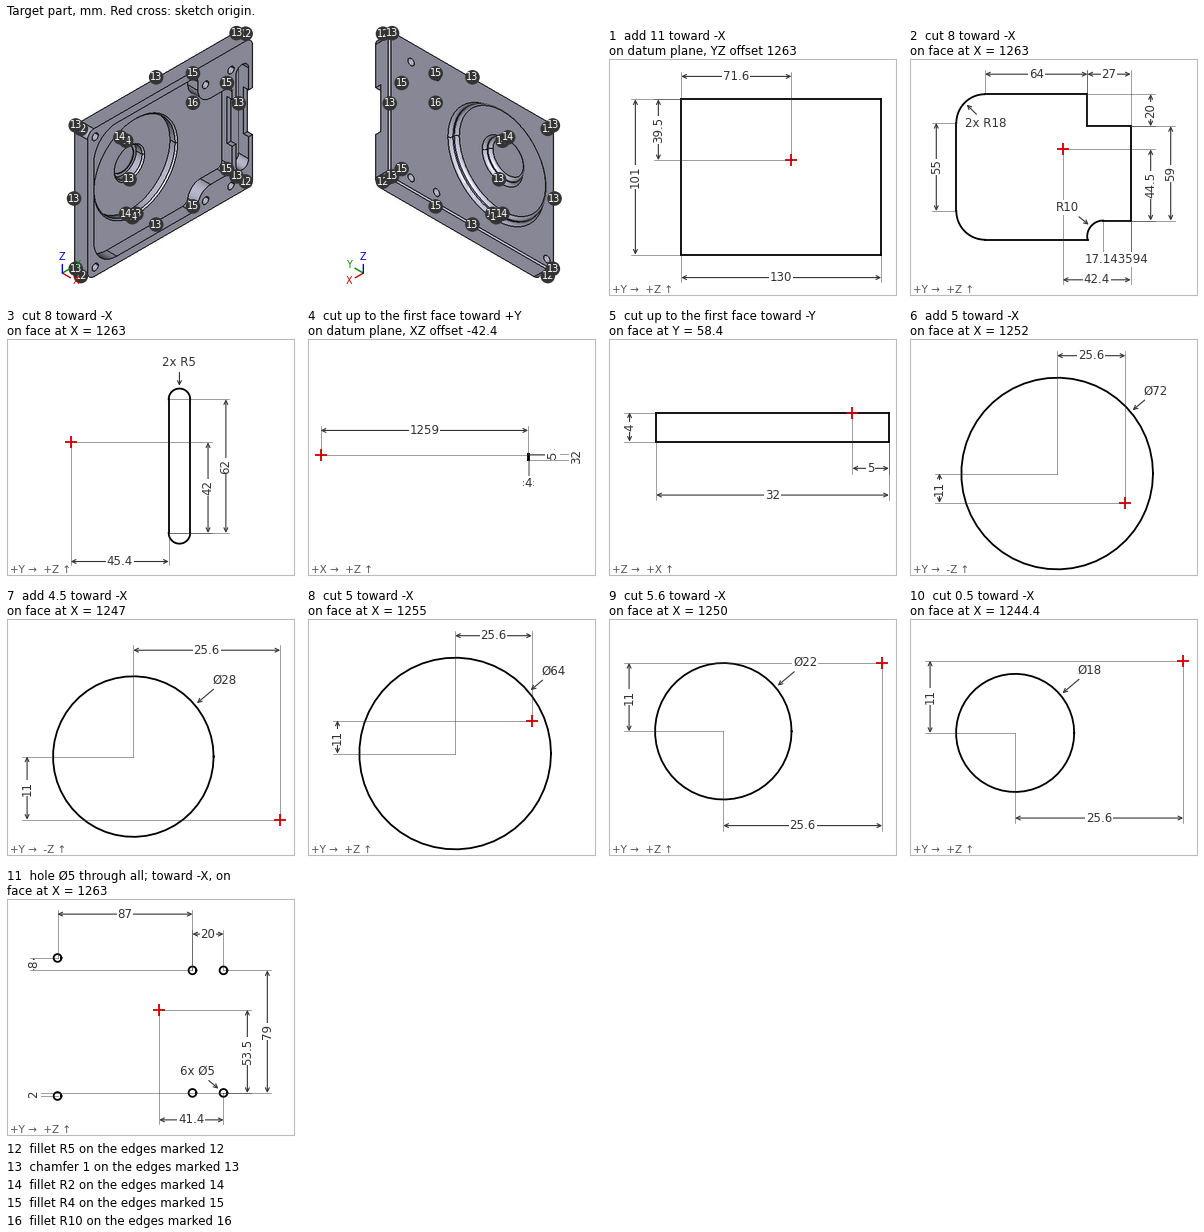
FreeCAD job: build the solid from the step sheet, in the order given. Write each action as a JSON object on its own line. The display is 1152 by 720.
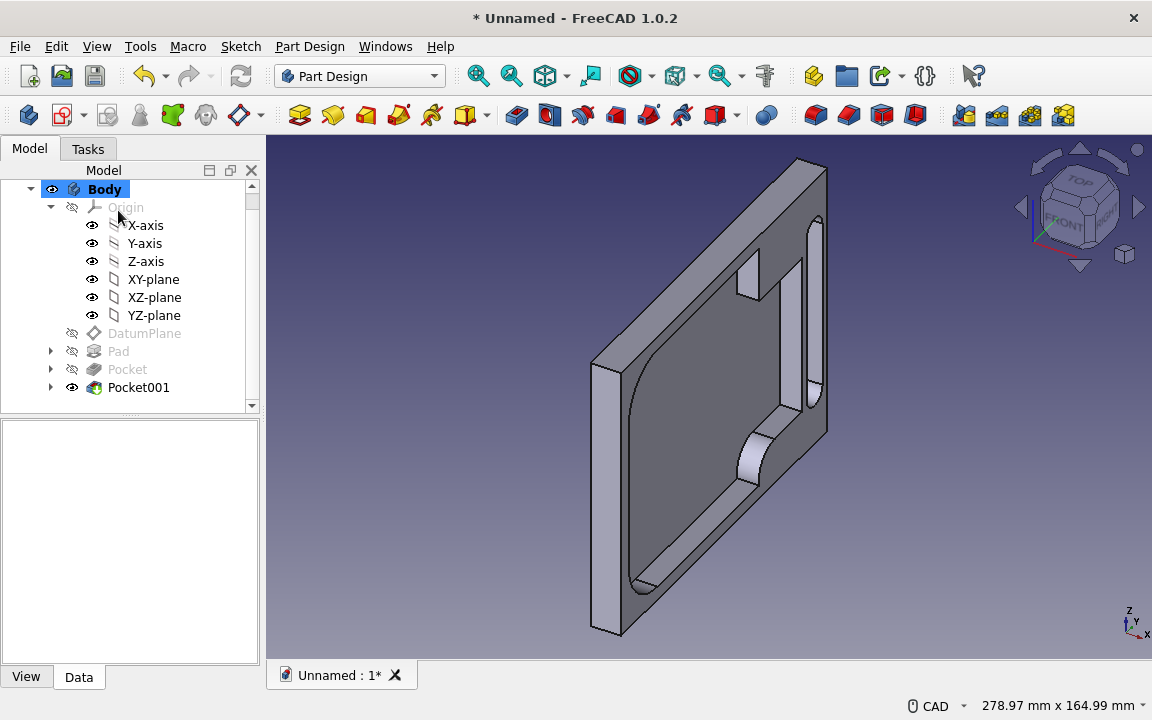
{"action": "left_click", "coordinate": [137, 297]}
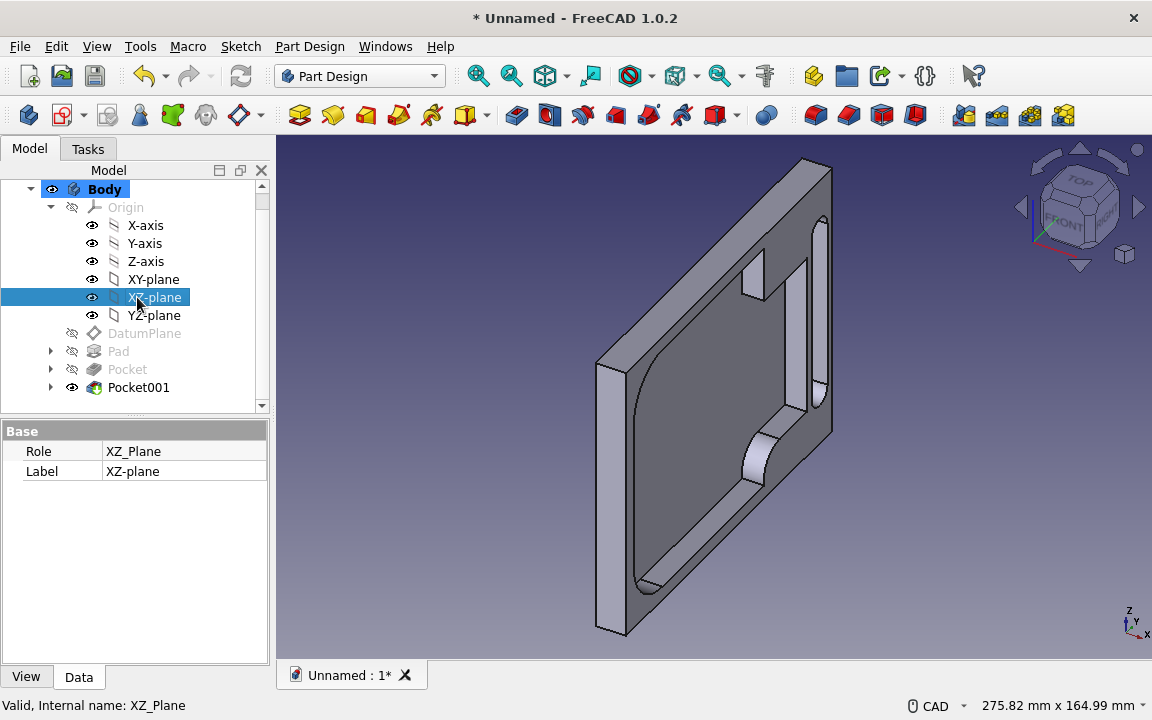
{"action": "left_click", "coordinate": [238, 116]}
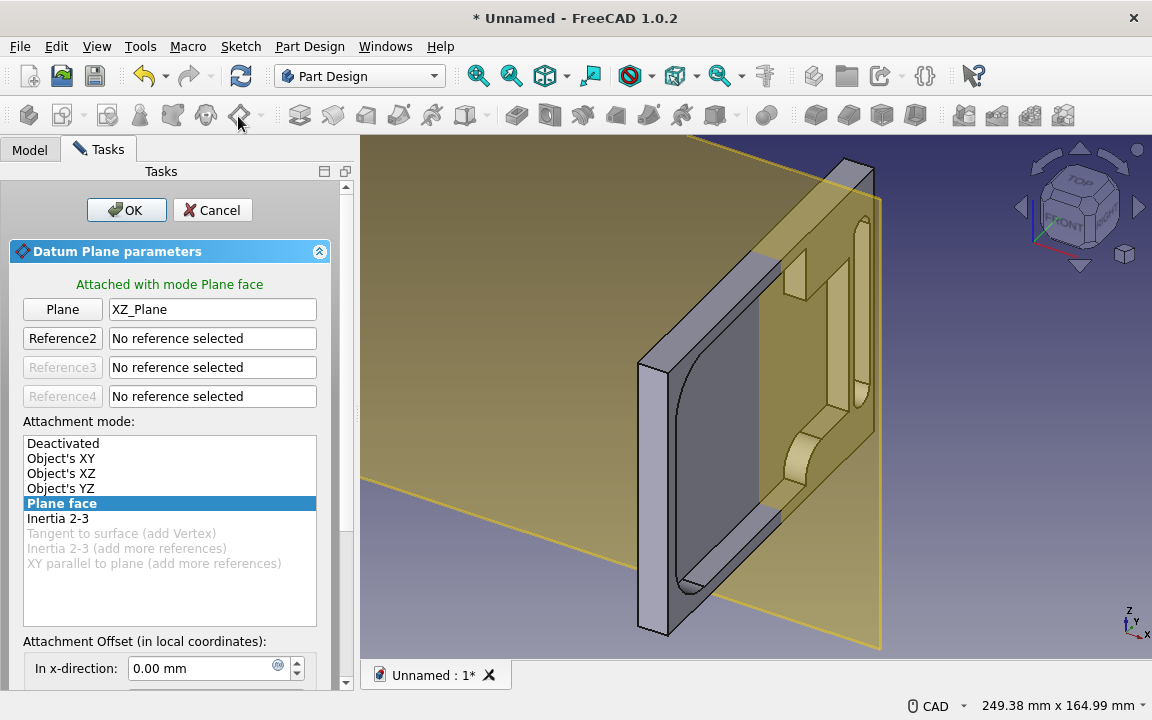
{"action": "scroll", "coordinate": [346, 436], "scroll_direction": "down", "scroll_amount": 2}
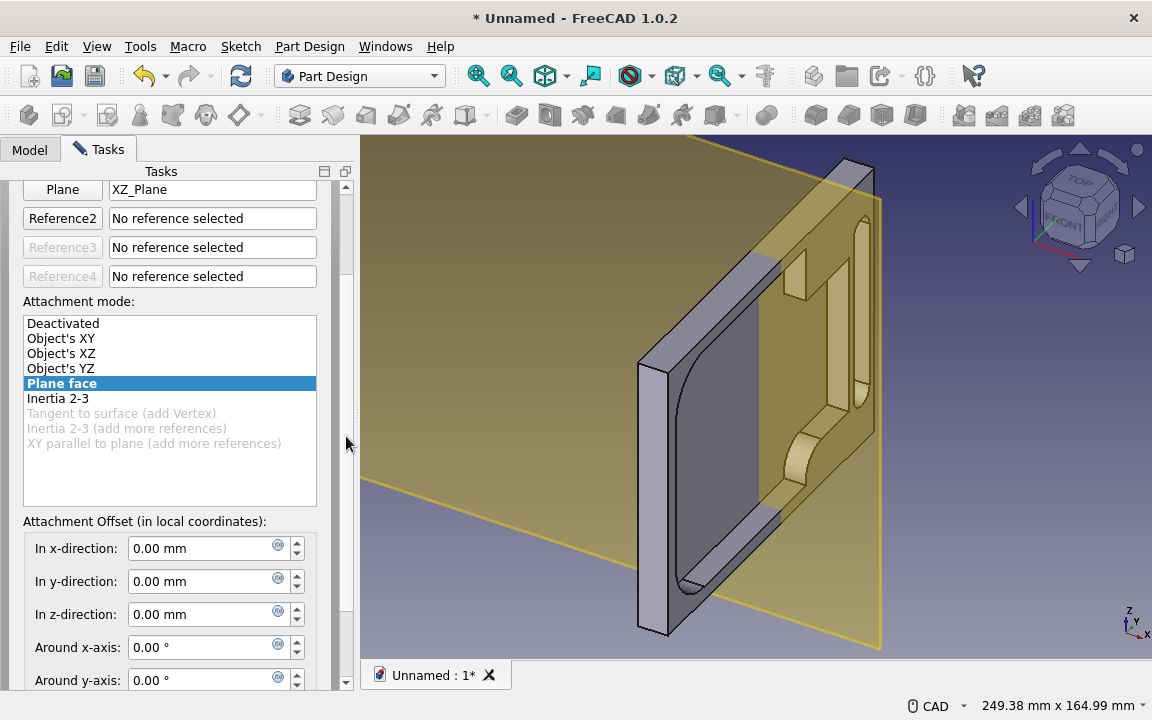
{"action": "triple_click", "coordinate": [210, 614]}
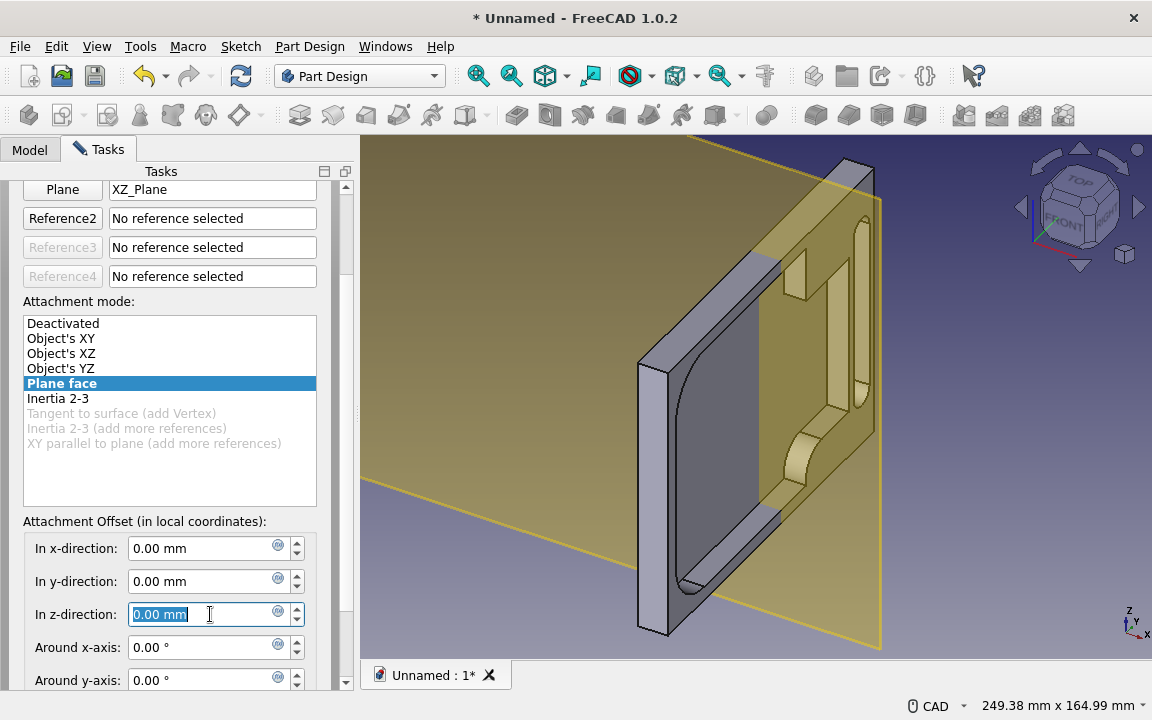
{"action": "type", "text": "-42.4"}
{"action": "key", "text": "Tab"}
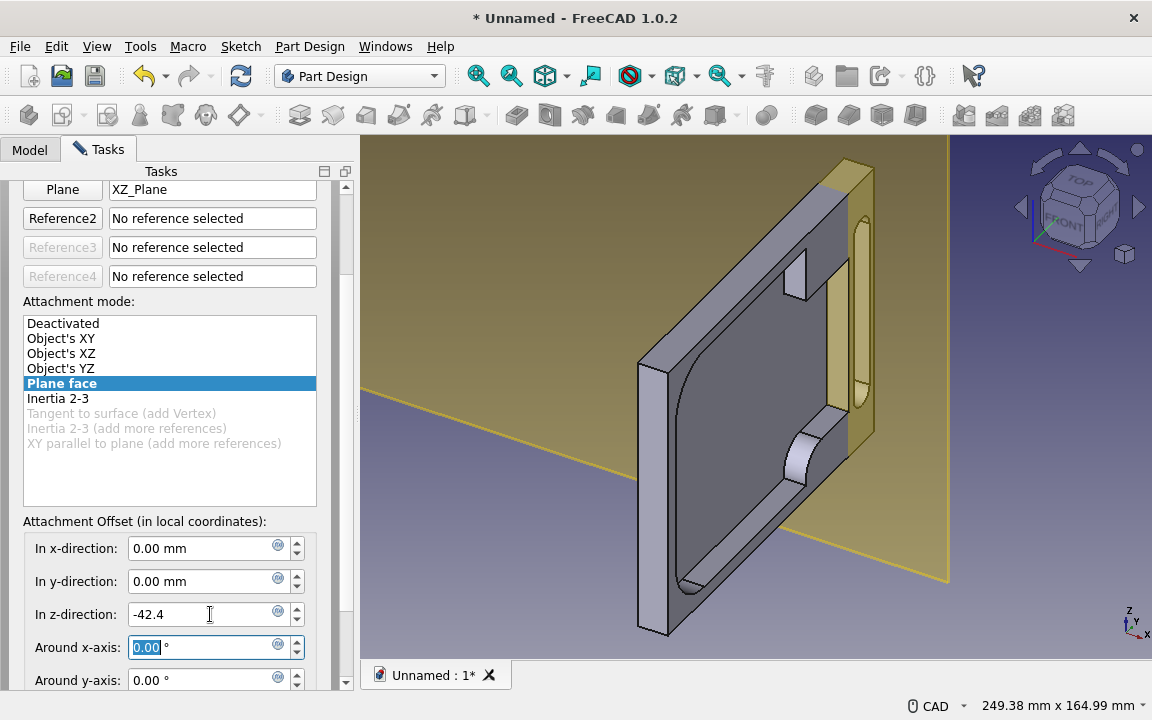
{"action": "scroll", "coordinate": [346, 436], "scroll_direction": "up", "scroll_amount": 3}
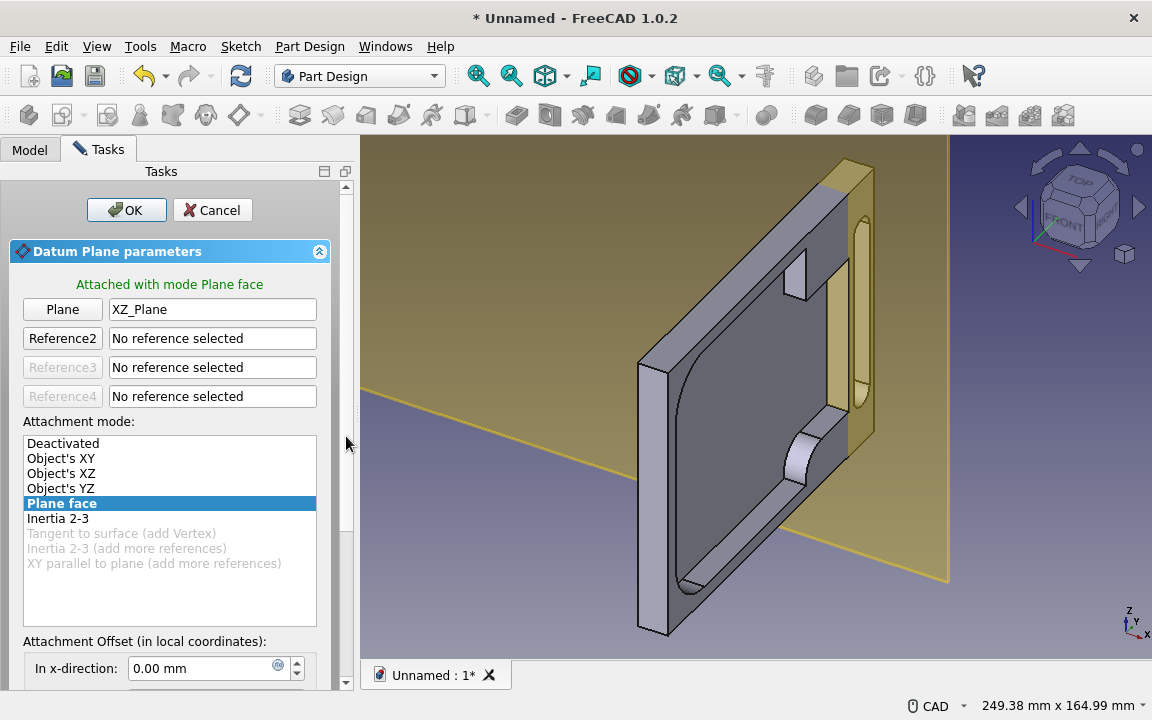
{"action": "left_click", "coordinate": [127, 210]}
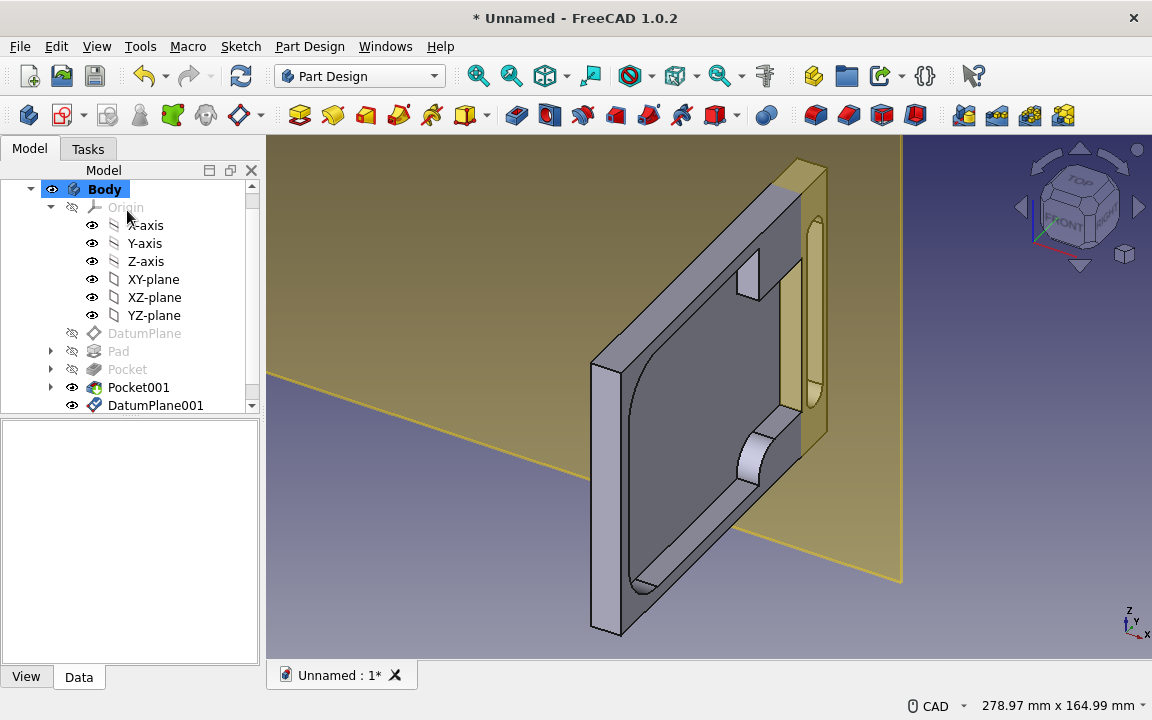
{"action": "left_click", "coordinate": [117, 405]}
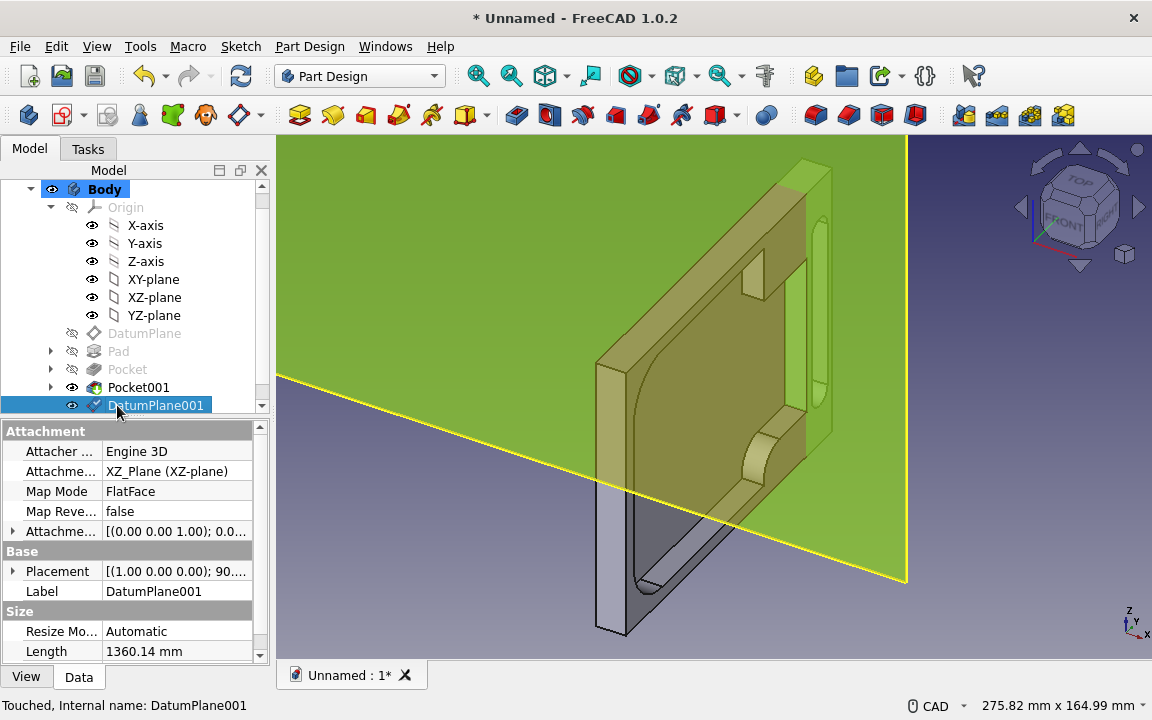
{"action": "left_click", "coordinate": [62, 116]}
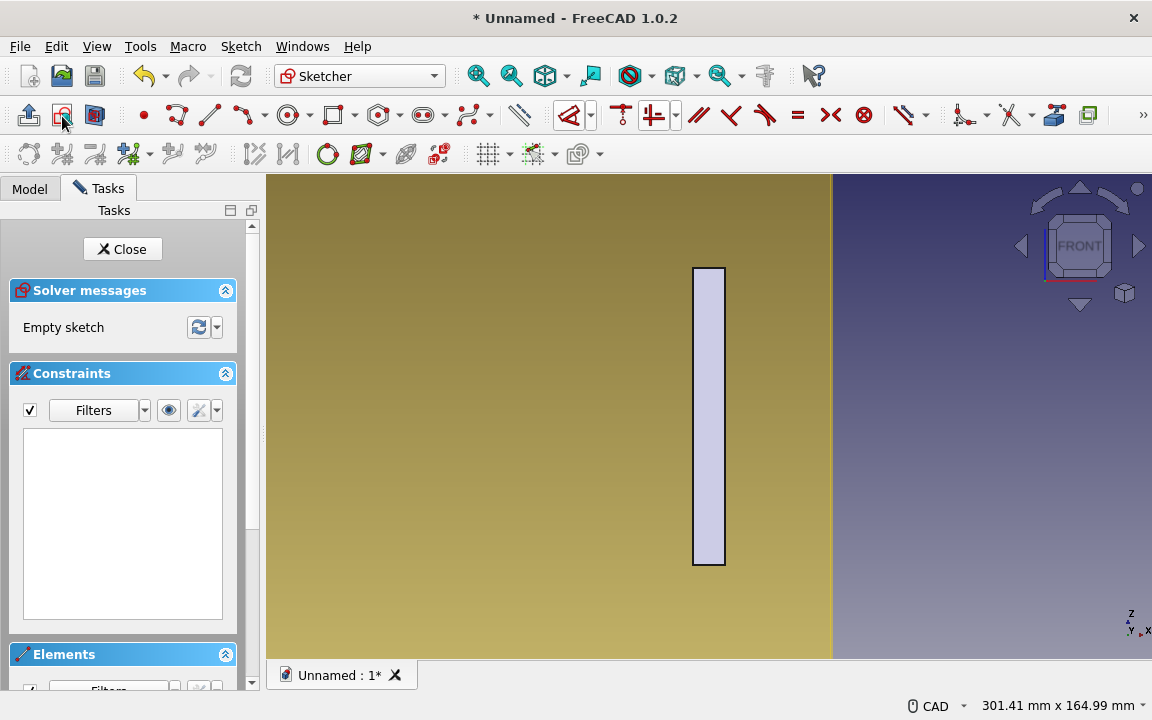
{"action": "left_click", "coordinate": [95, 116]}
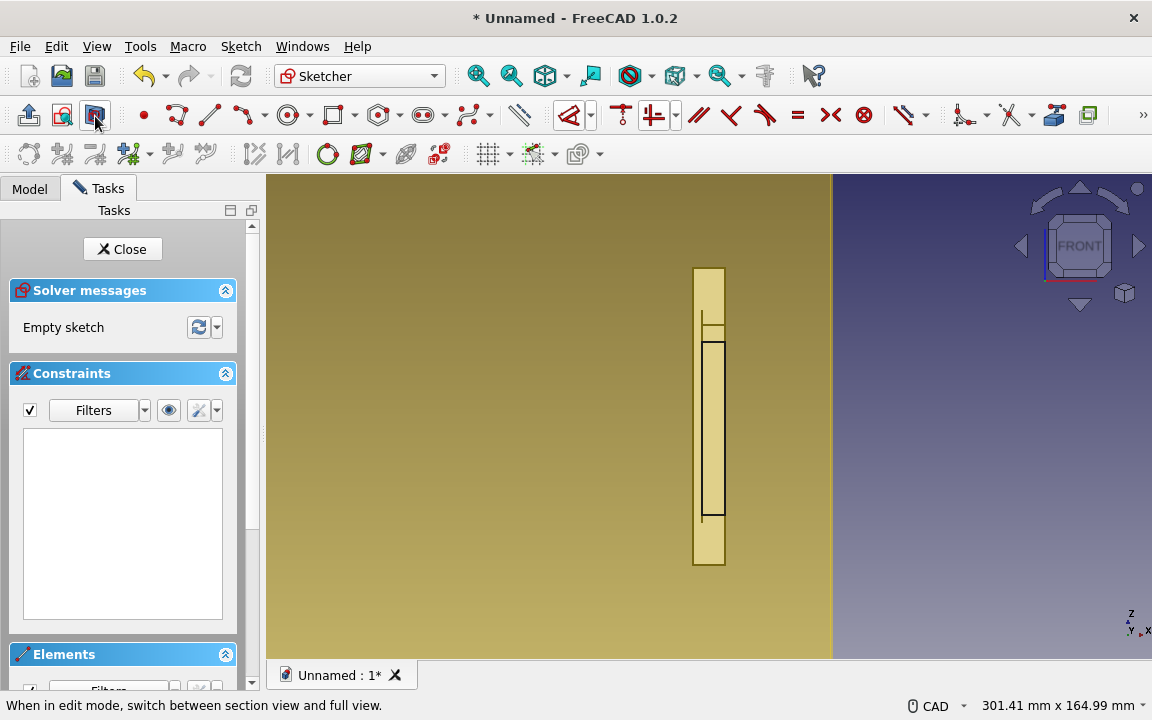
{"action": "scroll", "coordinate": [753, 417], "scroll_direction": "up", "scroll_amount": 6}